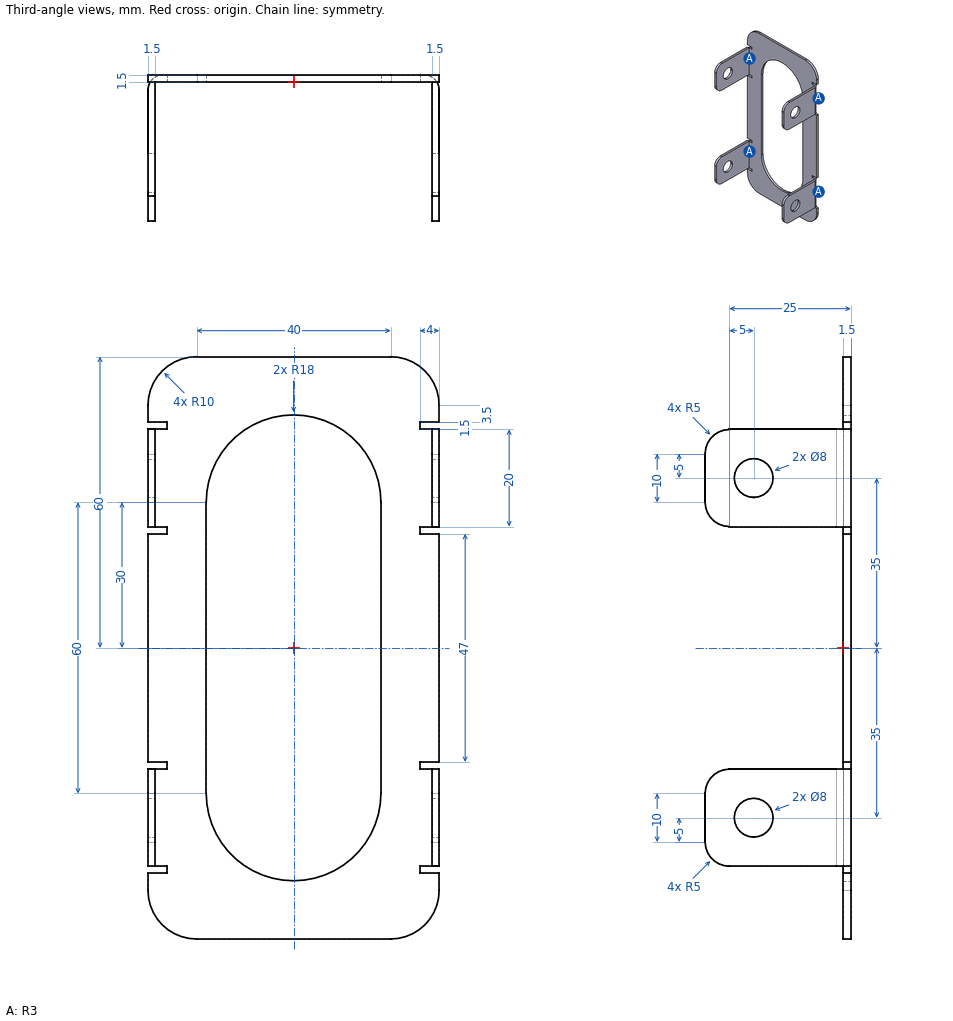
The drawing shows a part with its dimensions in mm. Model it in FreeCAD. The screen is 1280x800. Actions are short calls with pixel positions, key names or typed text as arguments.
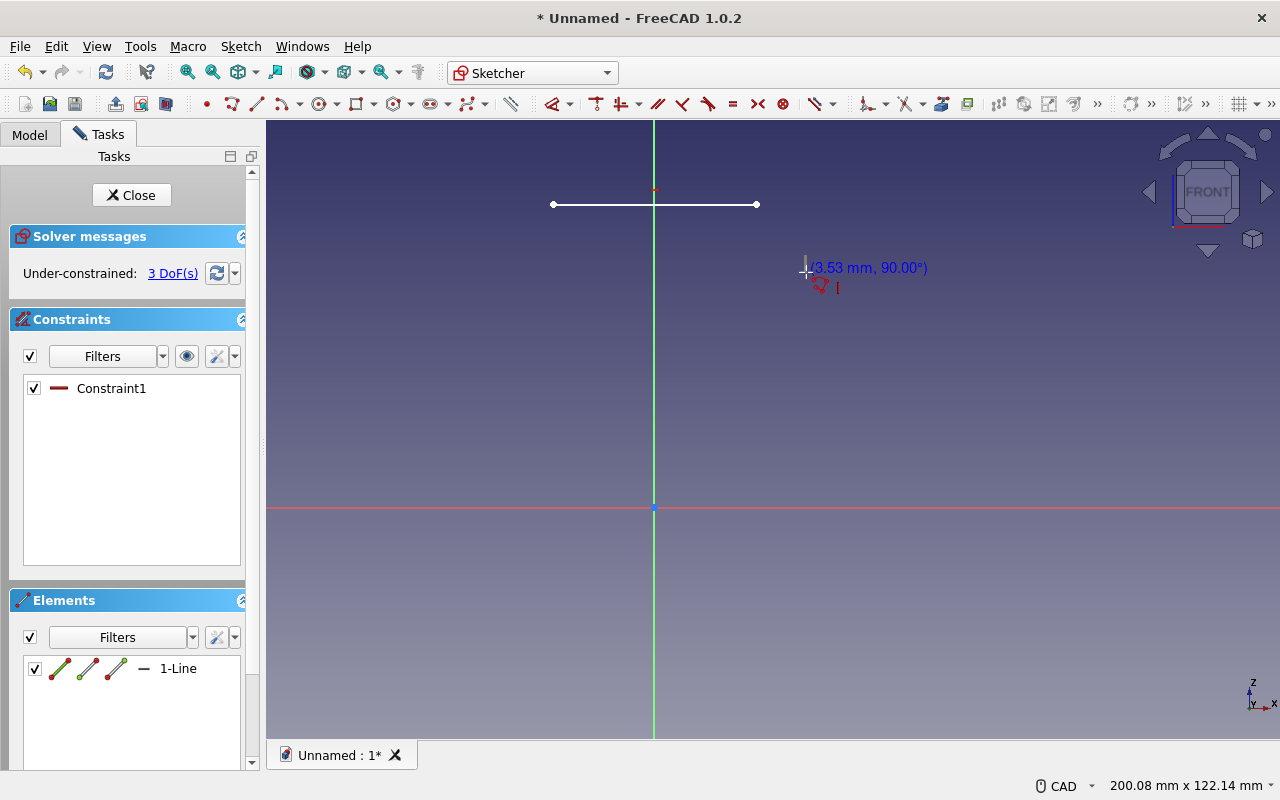
click(806, 272)
click(786, 272)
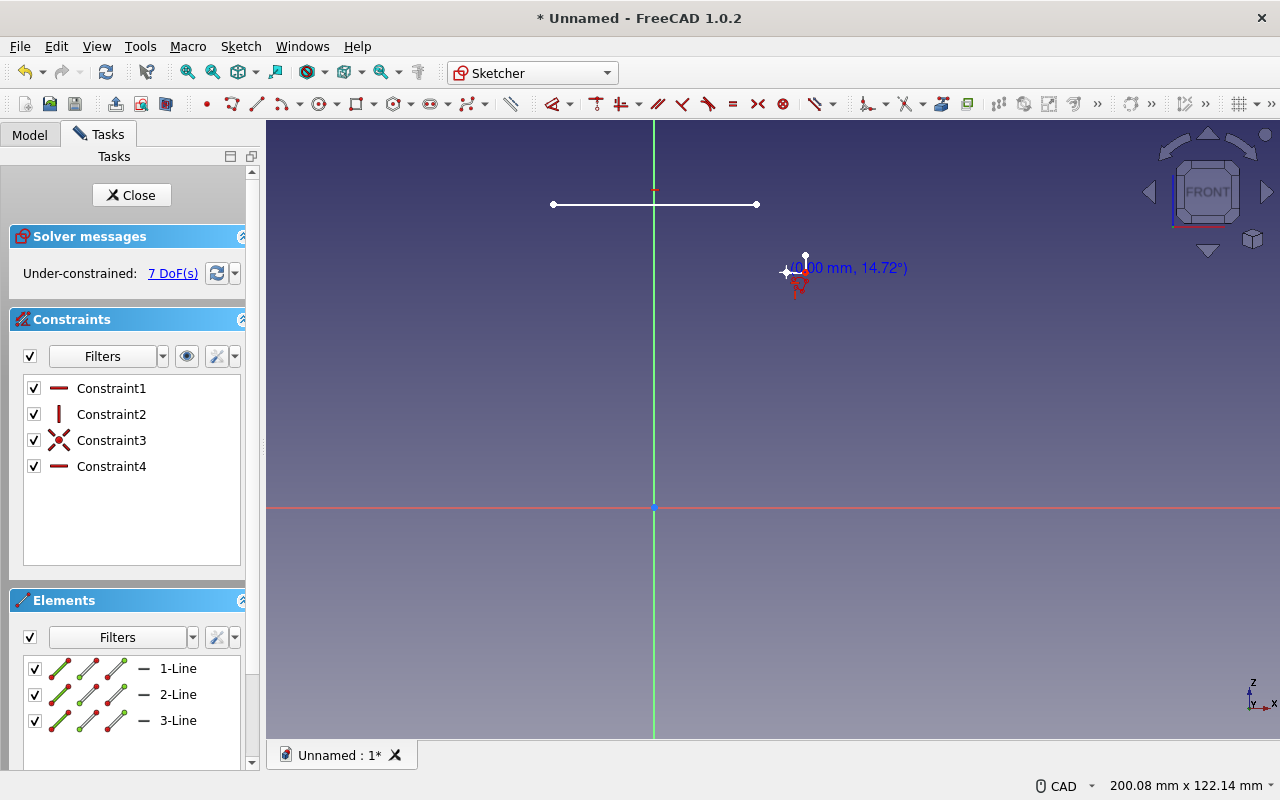
scroll(786, 279, up, 4)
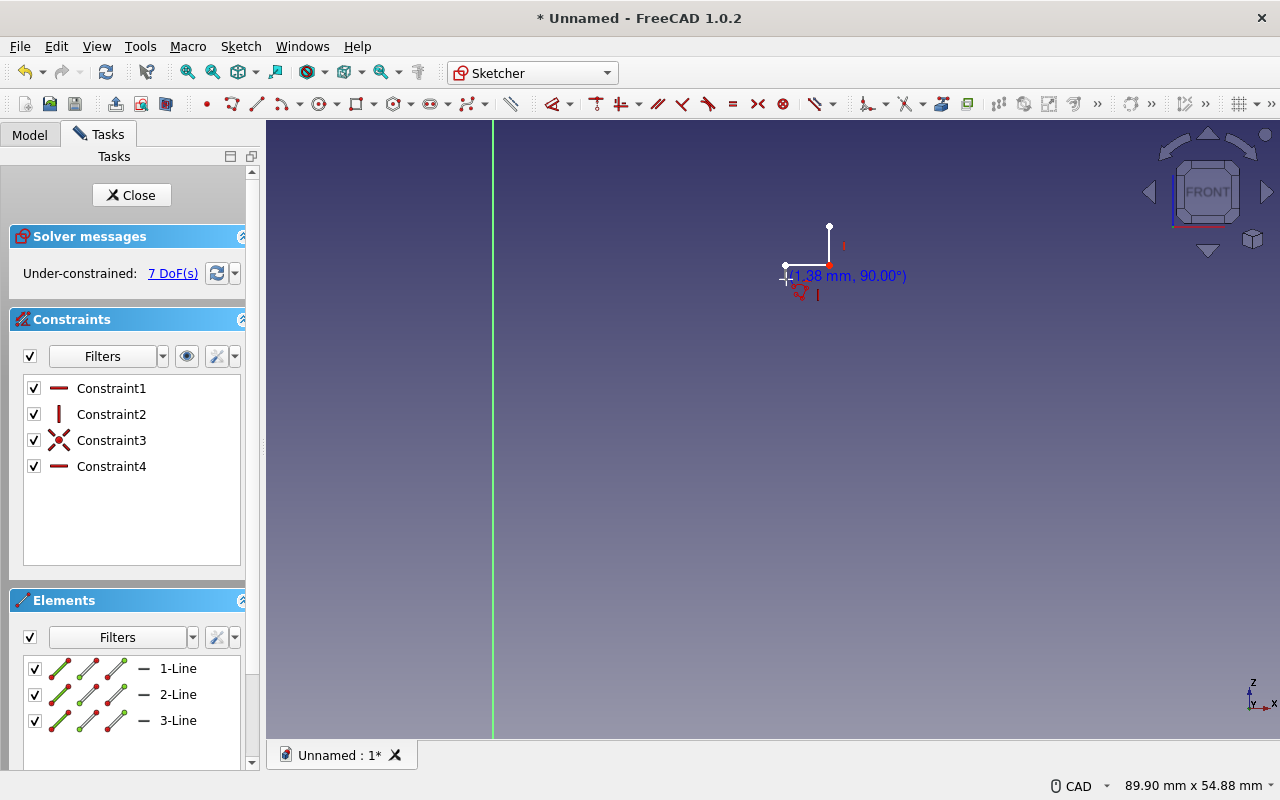
click(785, 280)
click(831, 280)
click(831, 505)
click(786, 505)
click(786, 522)
click(831, 522)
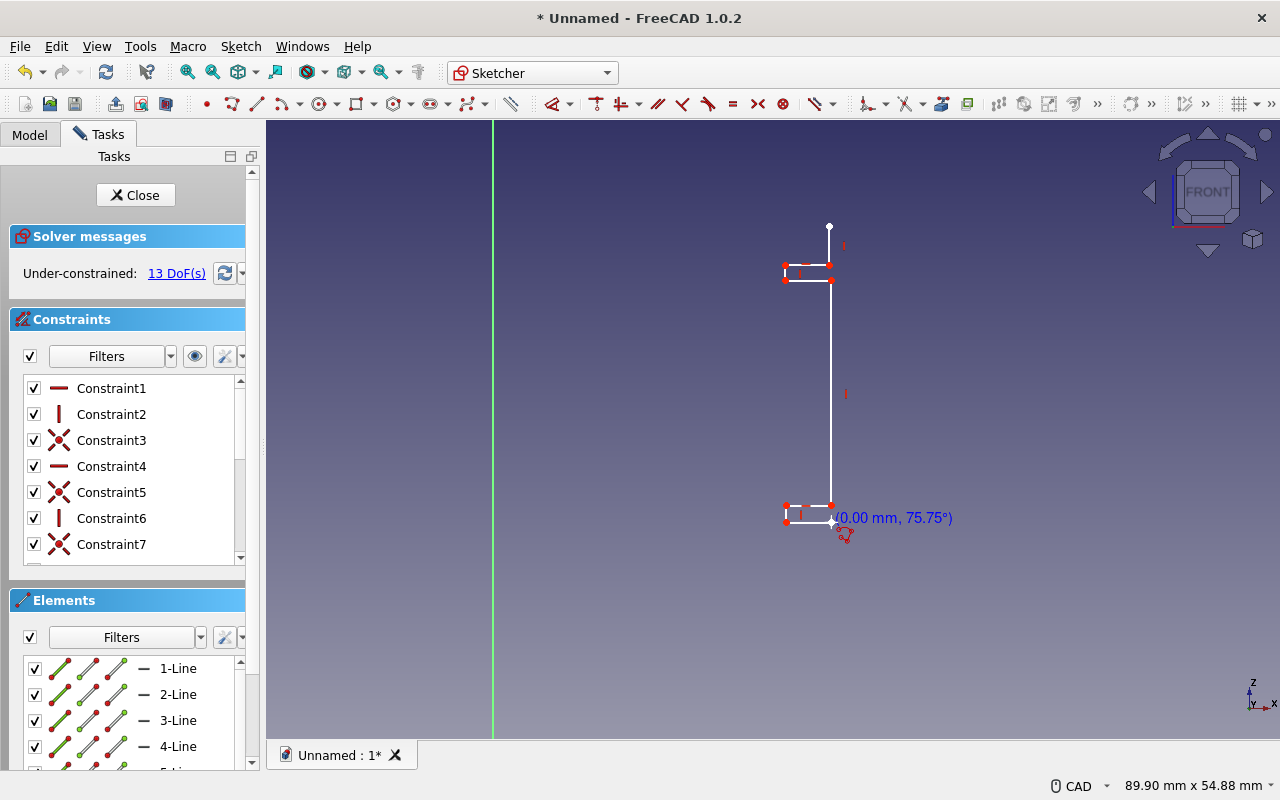
scroll(796, 275, down, 6)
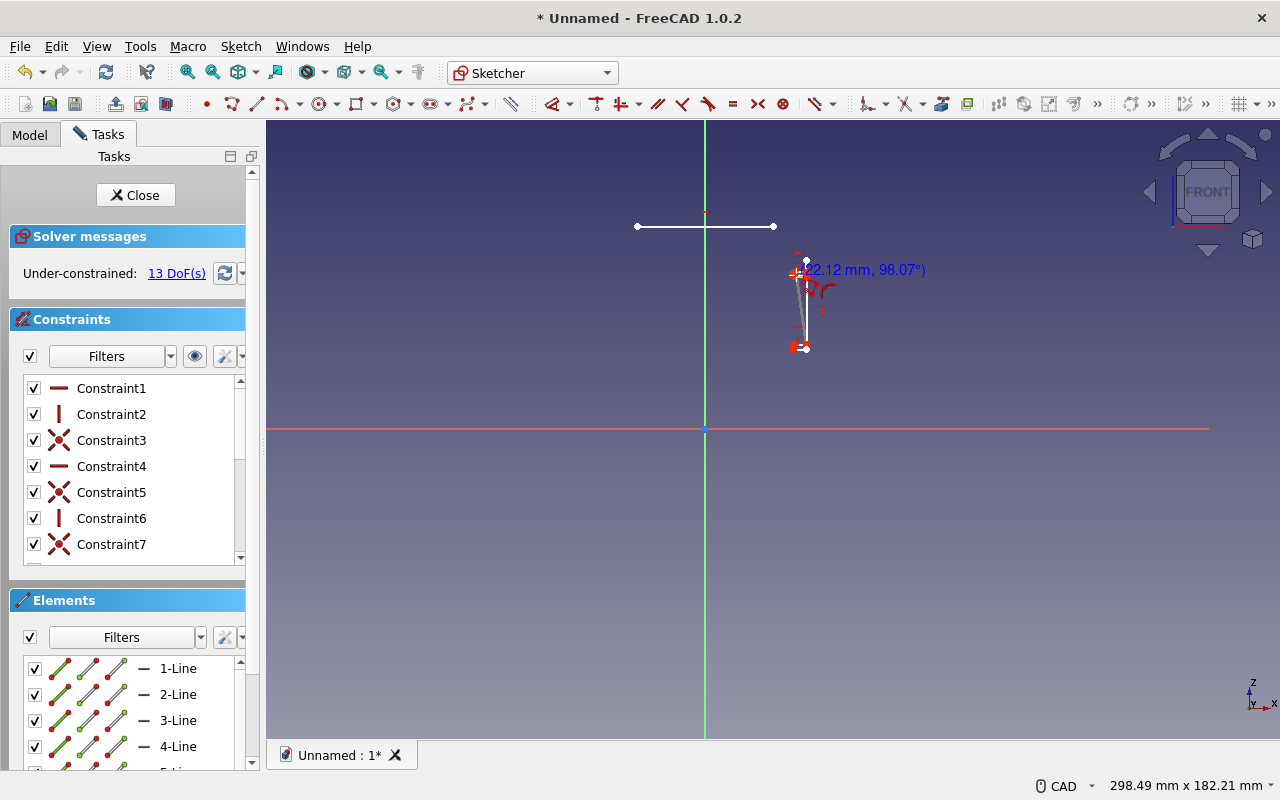
click(807, 509)
click(793, 509)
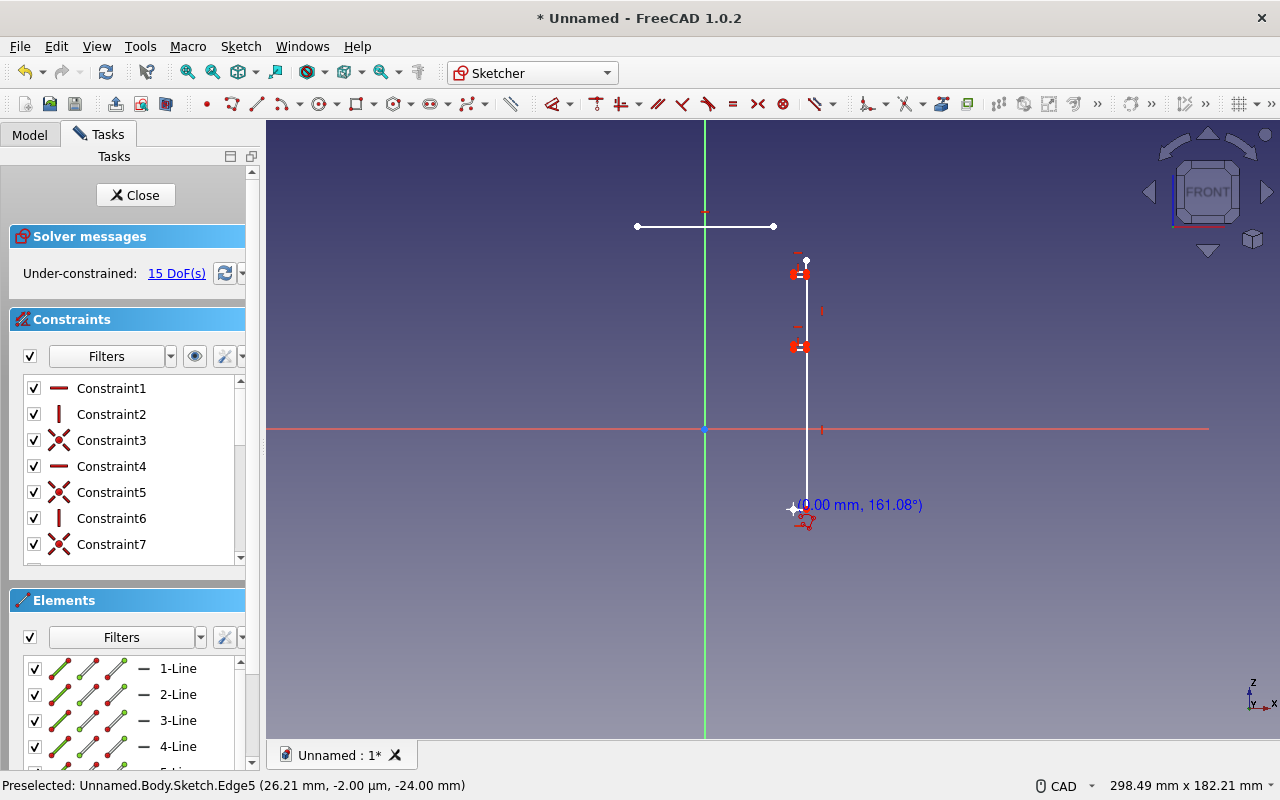
scroll(793, 514, up, 6)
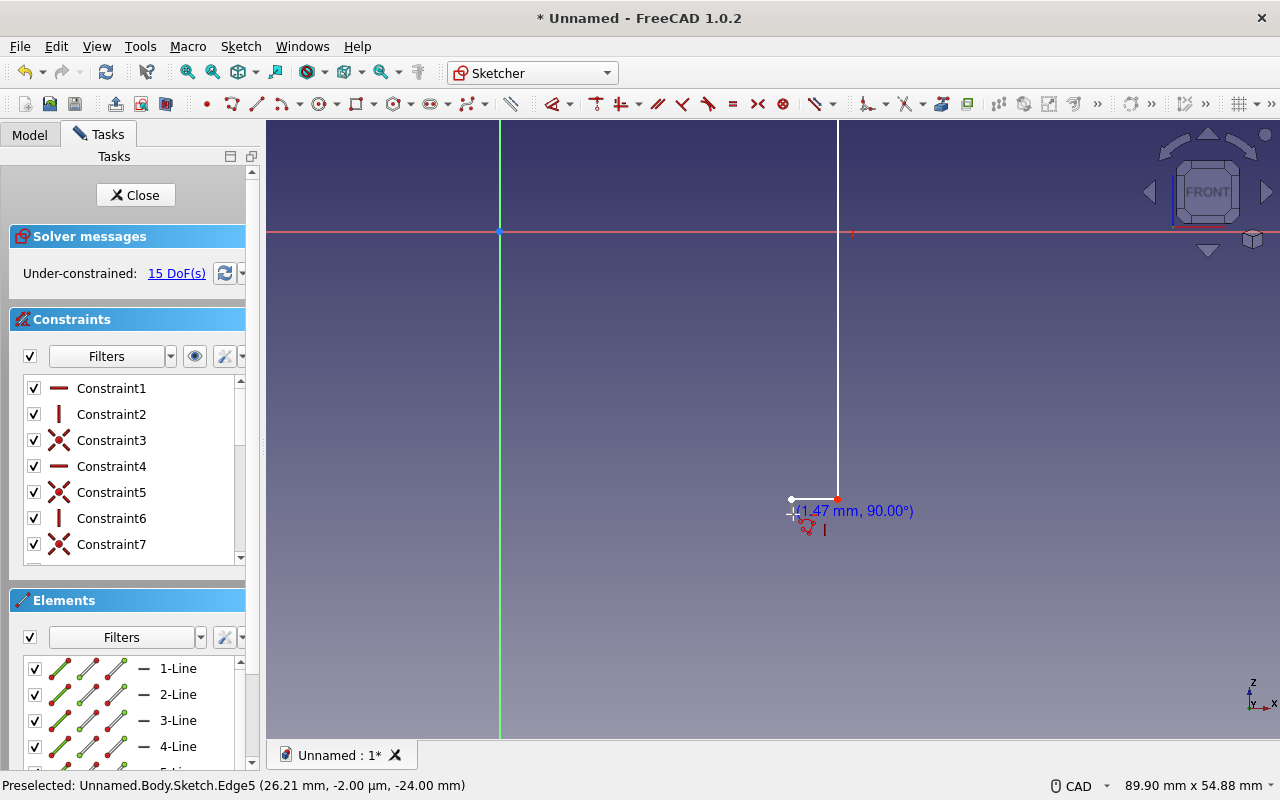
click(792, 514)
click(838, 514)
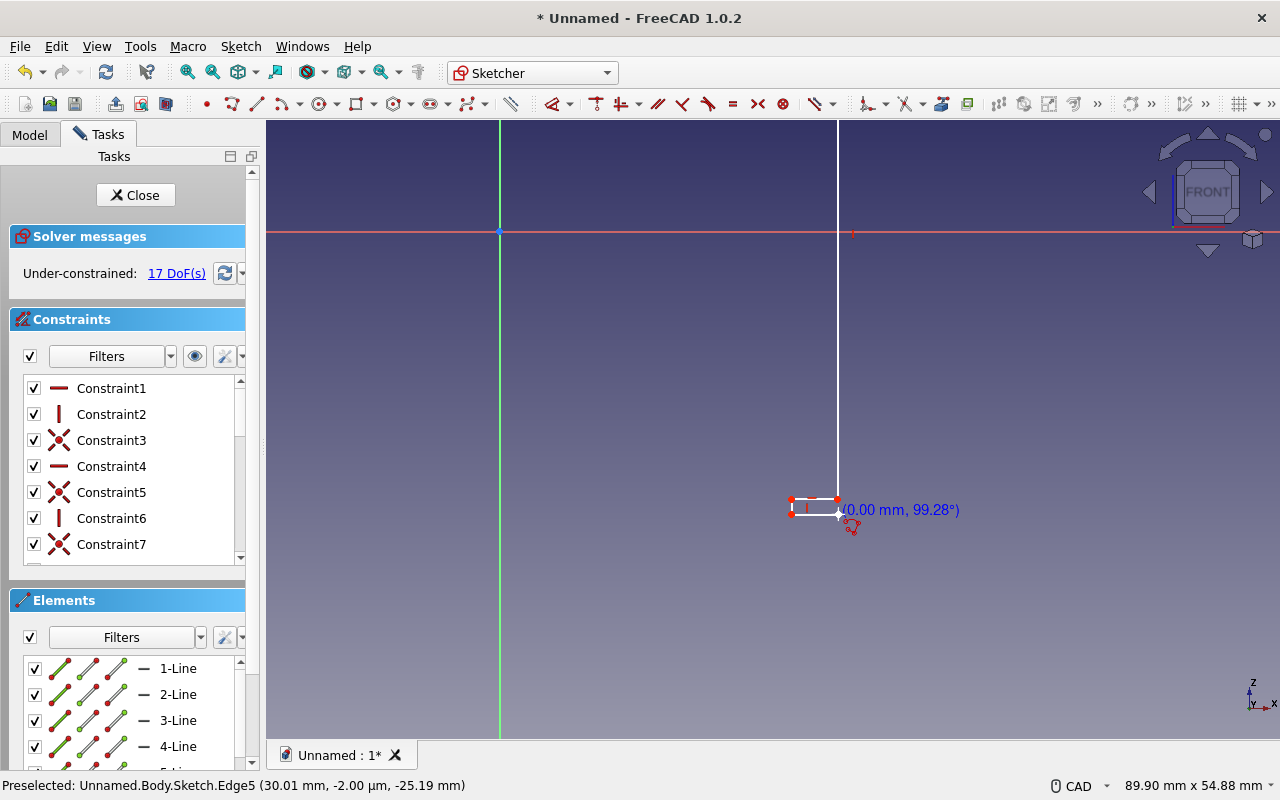
scroll(793, 515, down, 6)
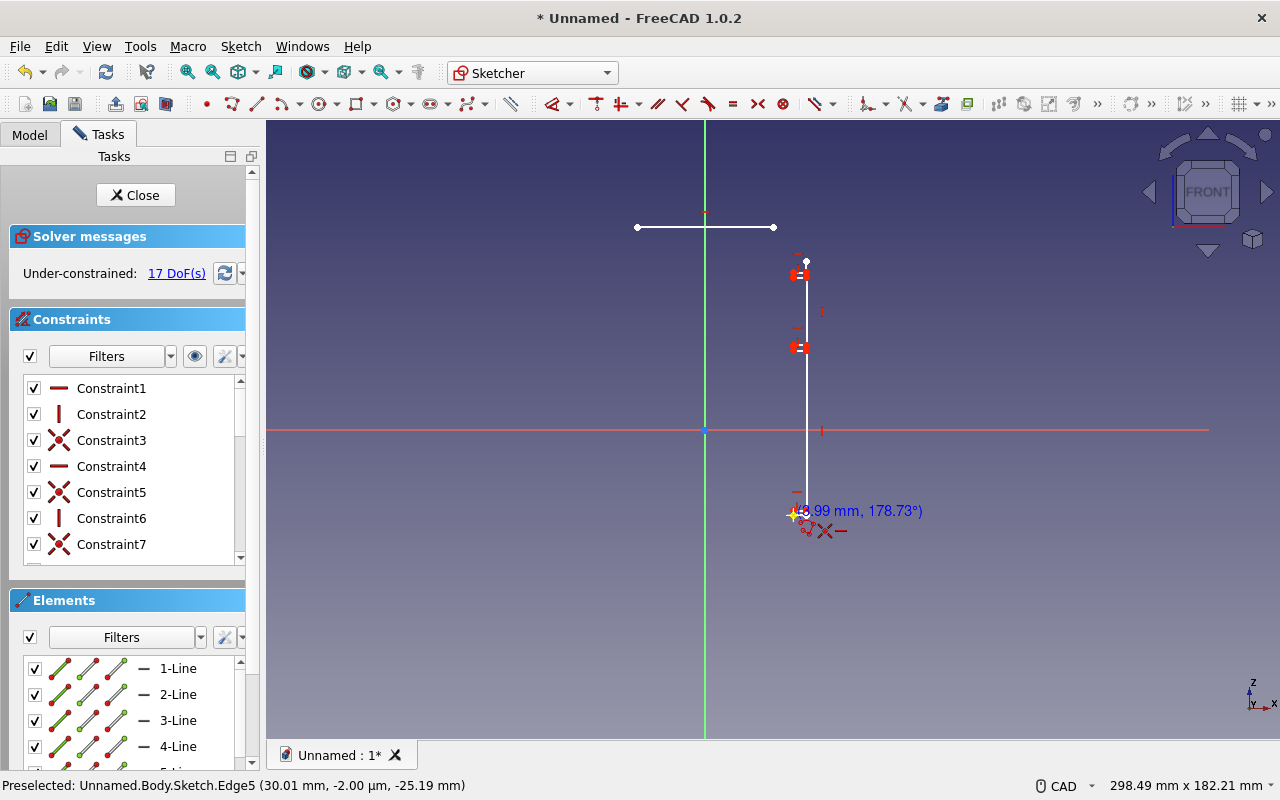
click(807, 583)
click(793, 583)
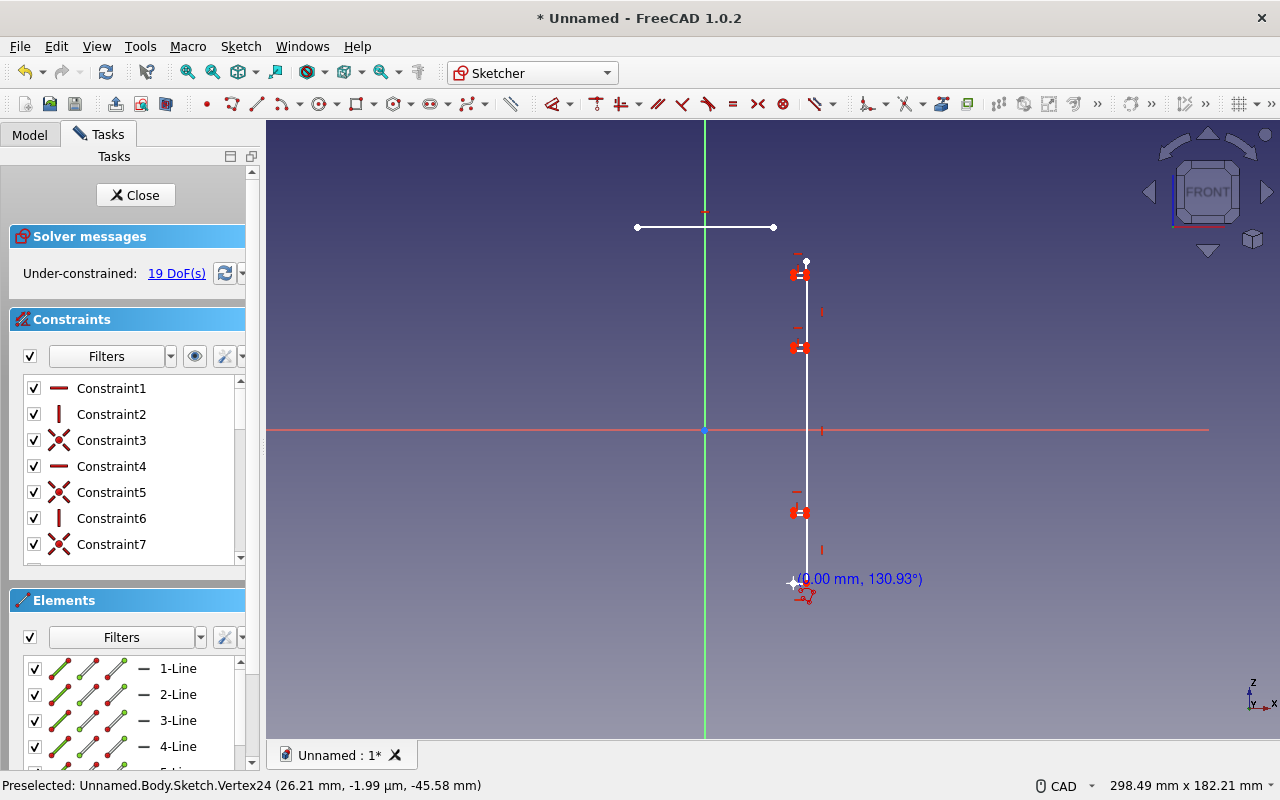
scroll(793, 588, up, 6)